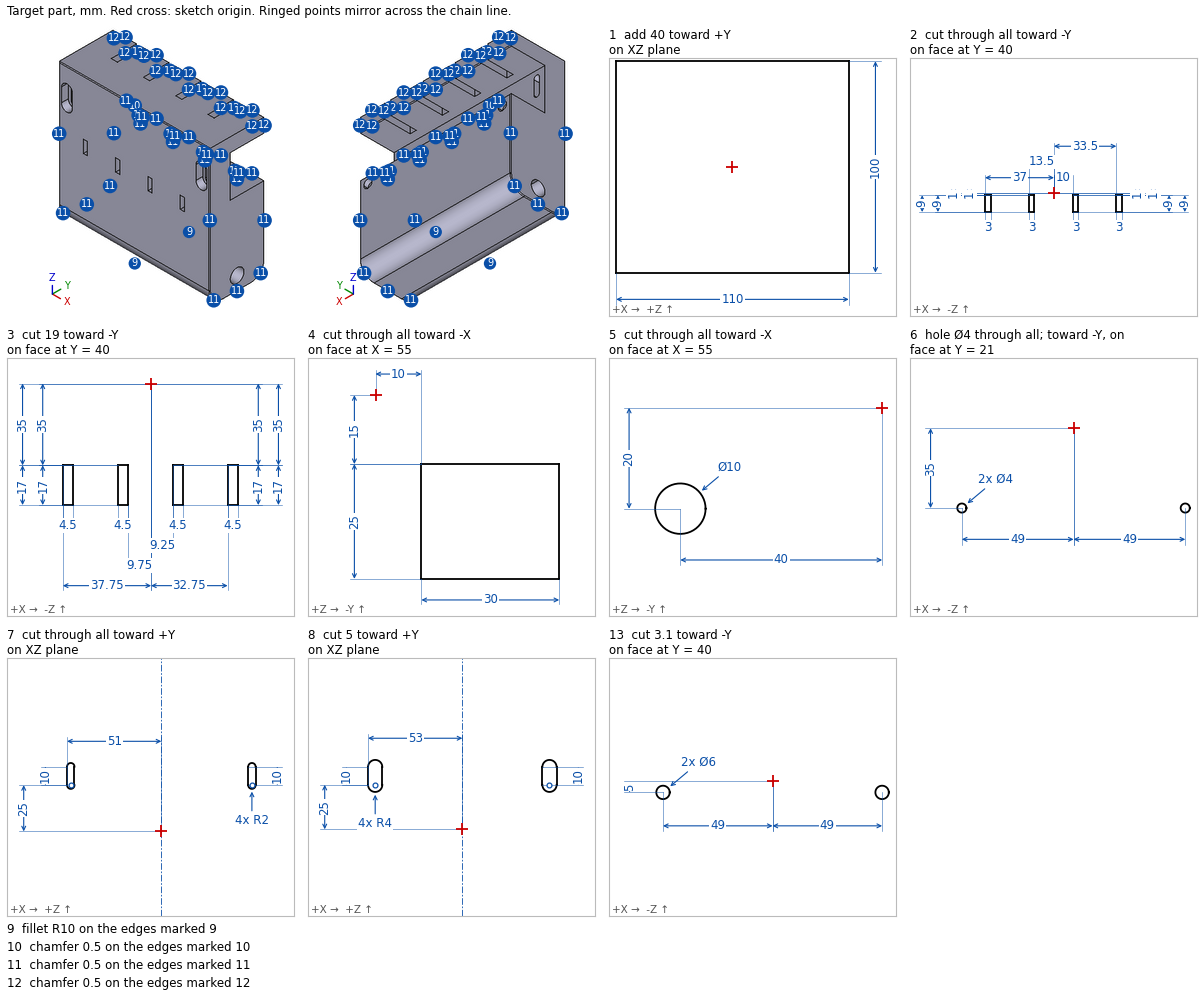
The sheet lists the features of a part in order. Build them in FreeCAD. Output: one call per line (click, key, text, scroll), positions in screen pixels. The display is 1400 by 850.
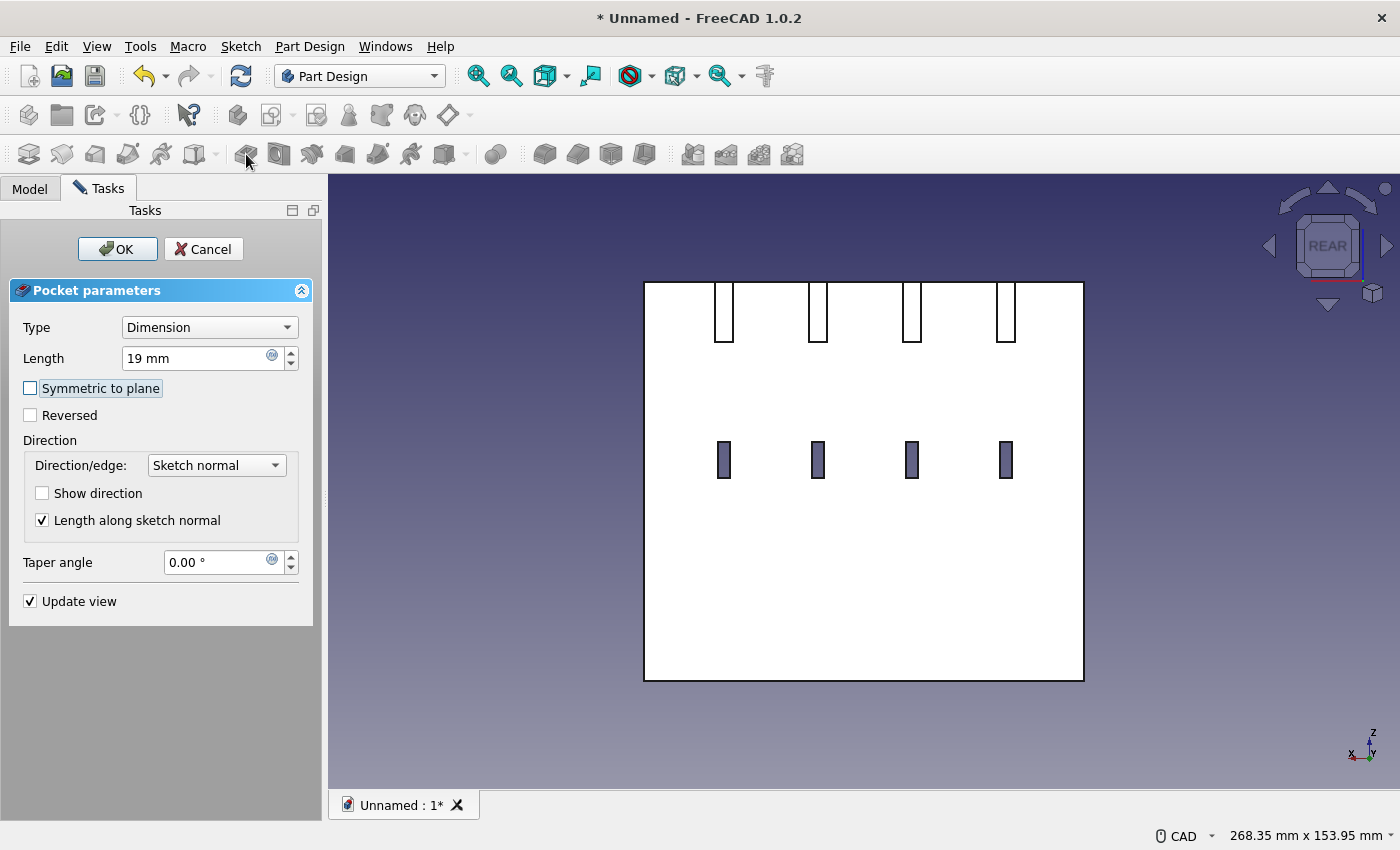
click(118, 249)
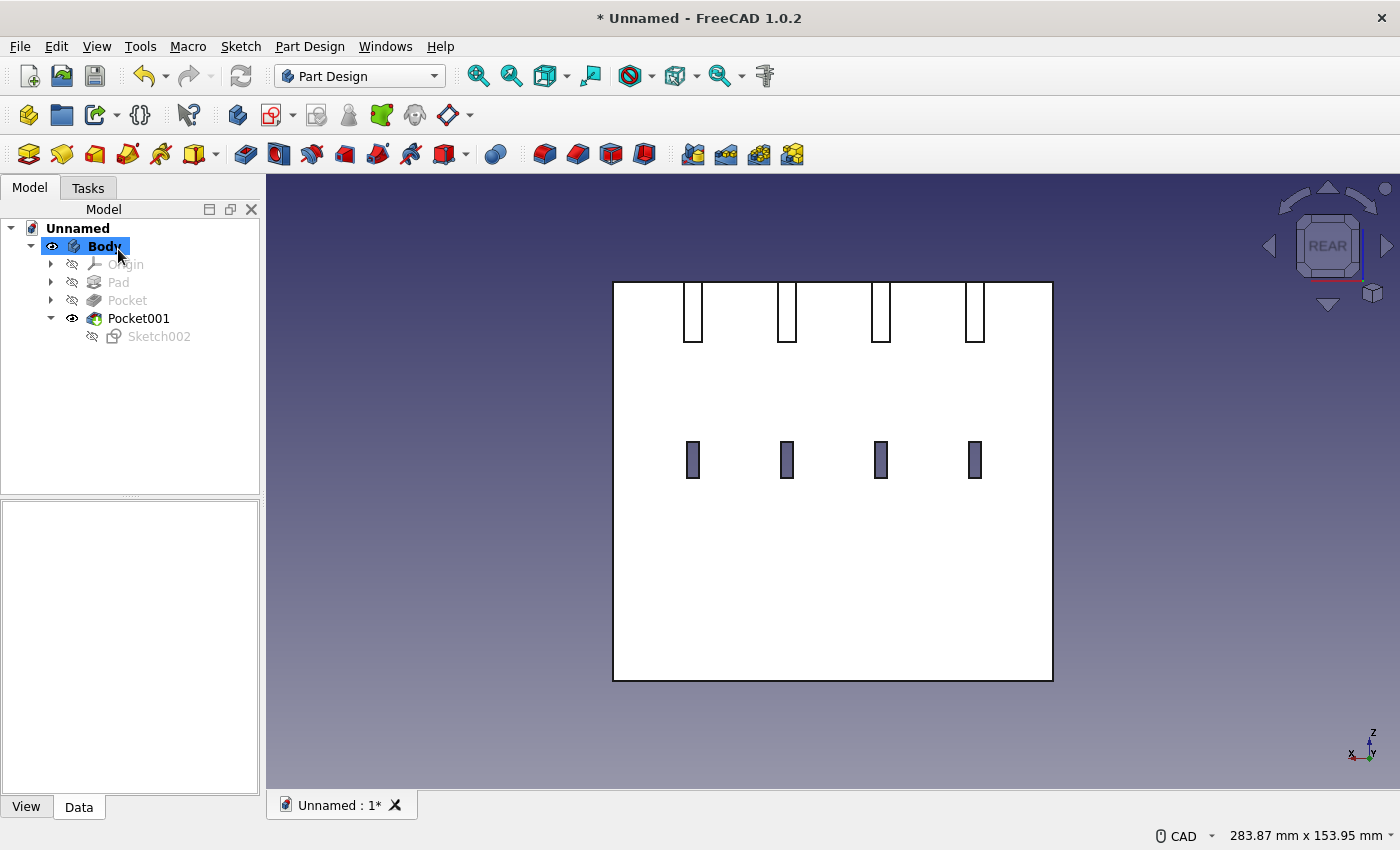
key(0)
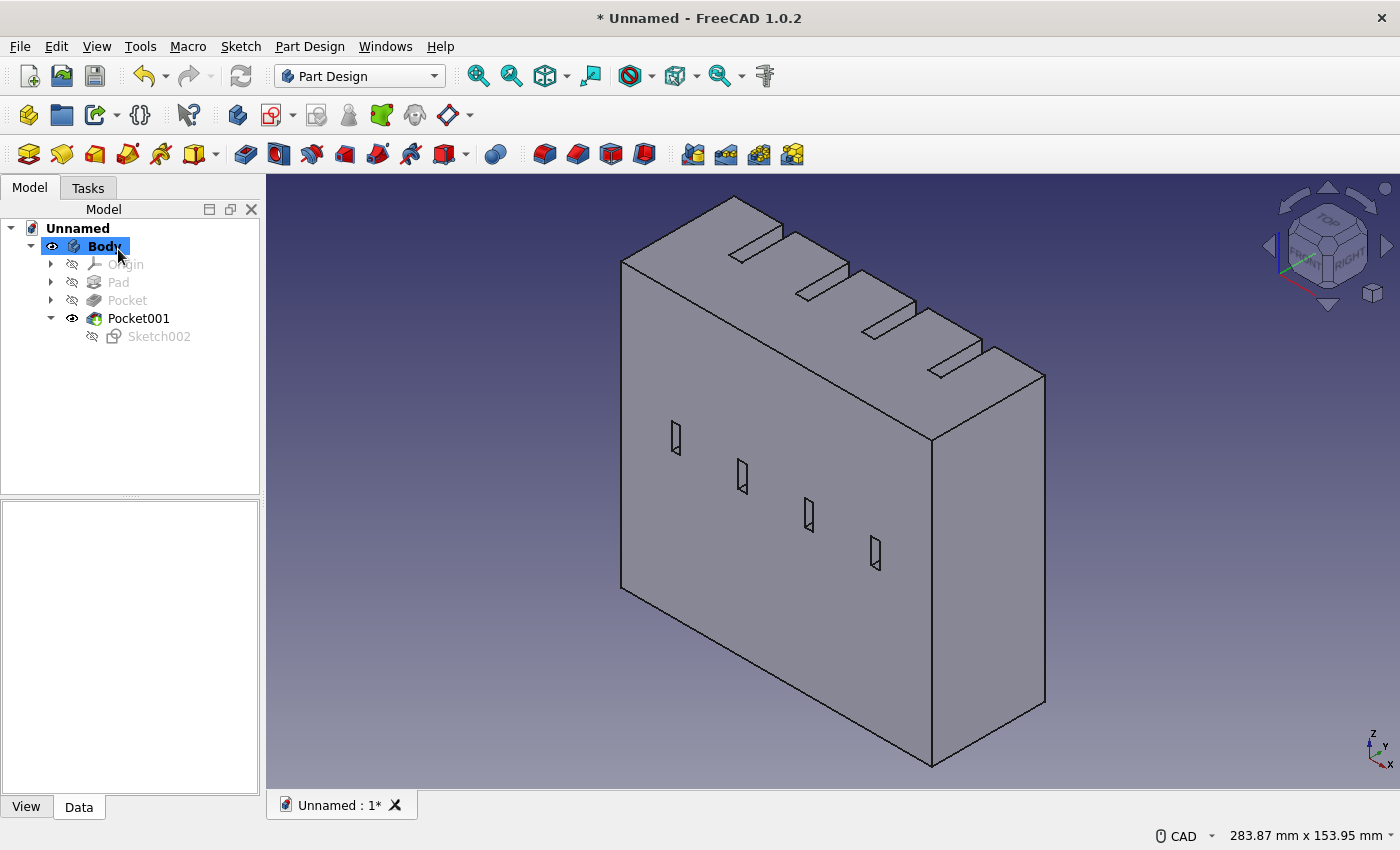
click(988, 570)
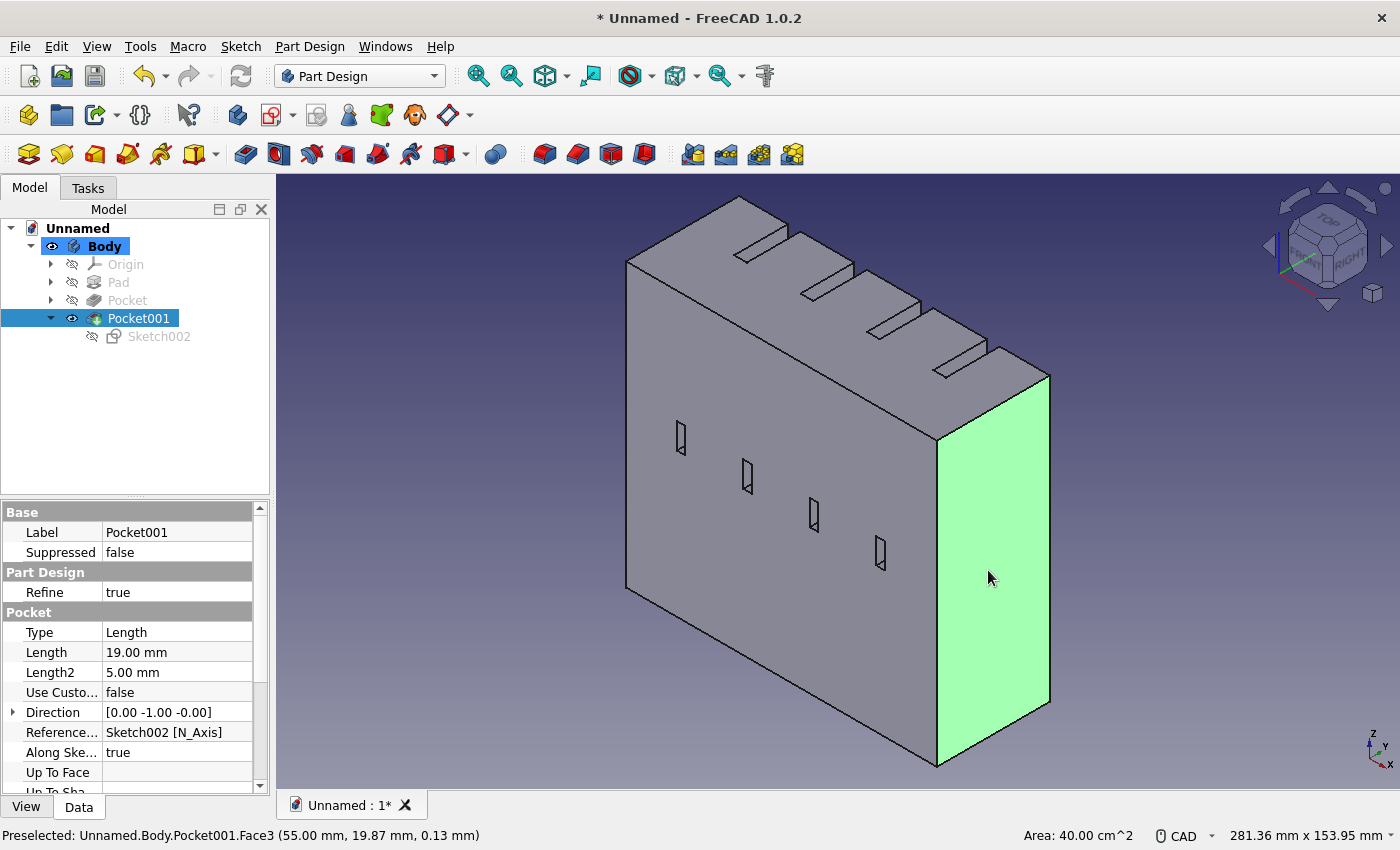
click(270, 116)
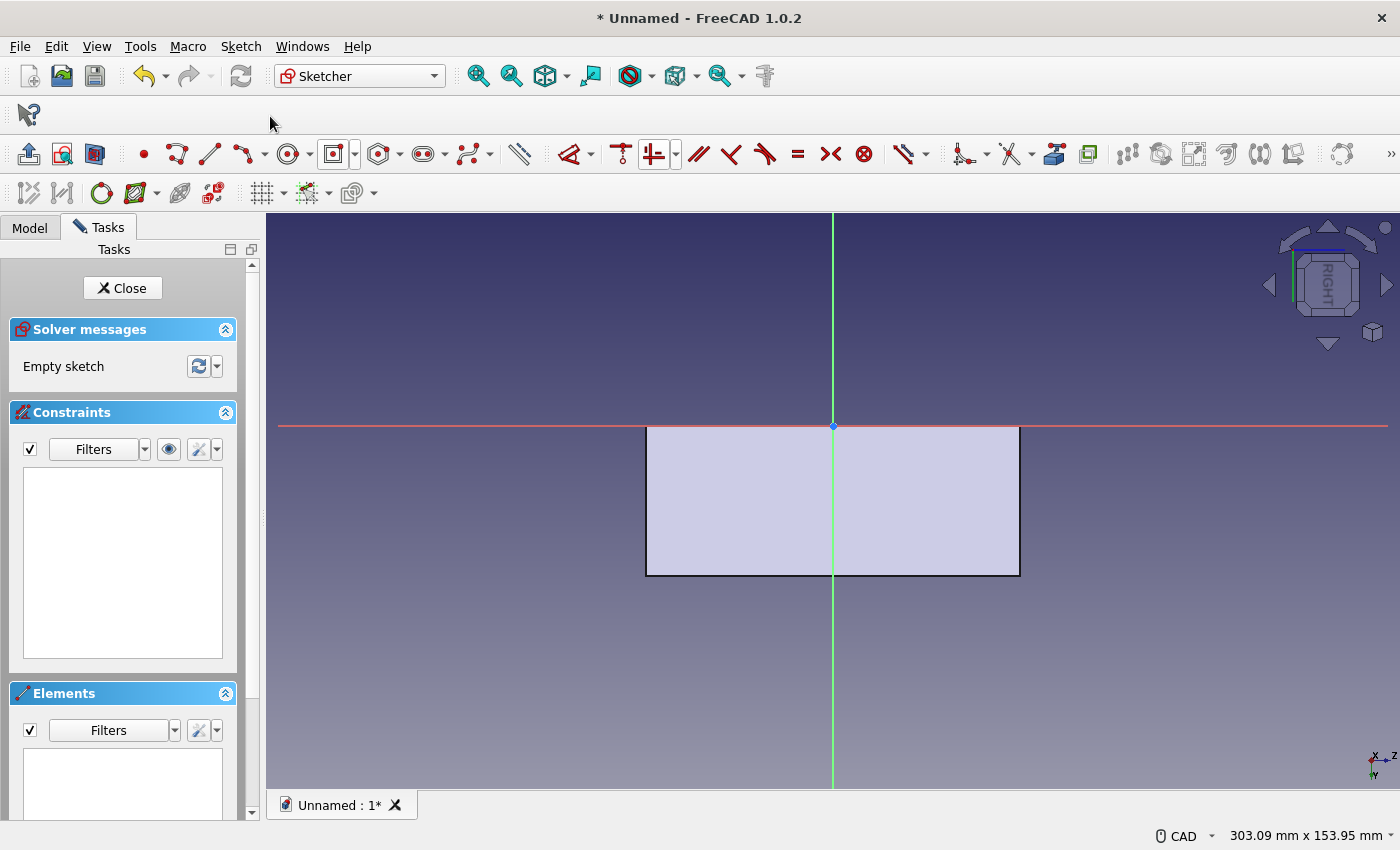
scroll(1025, 501, up, 4)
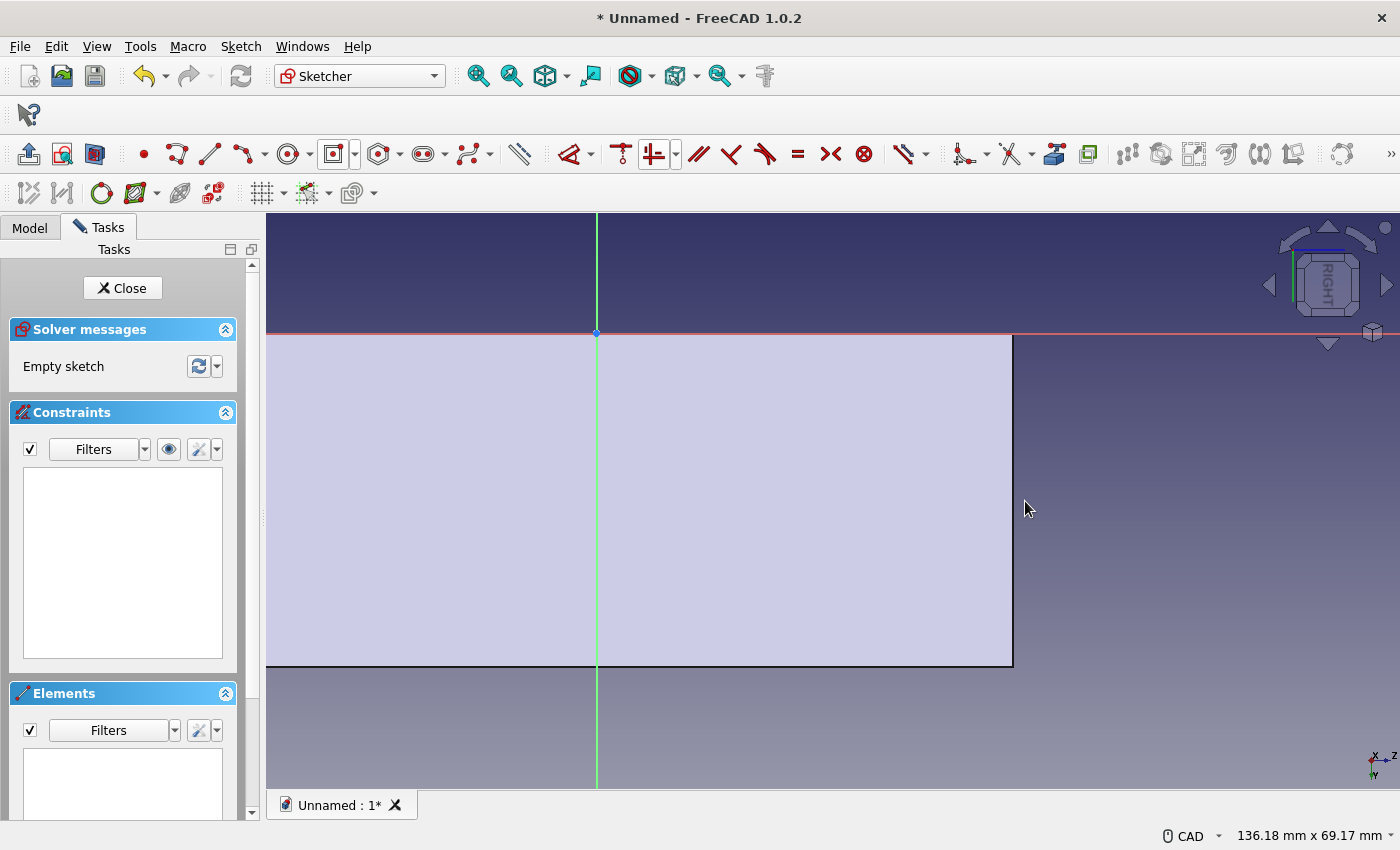
key(g)
key(r)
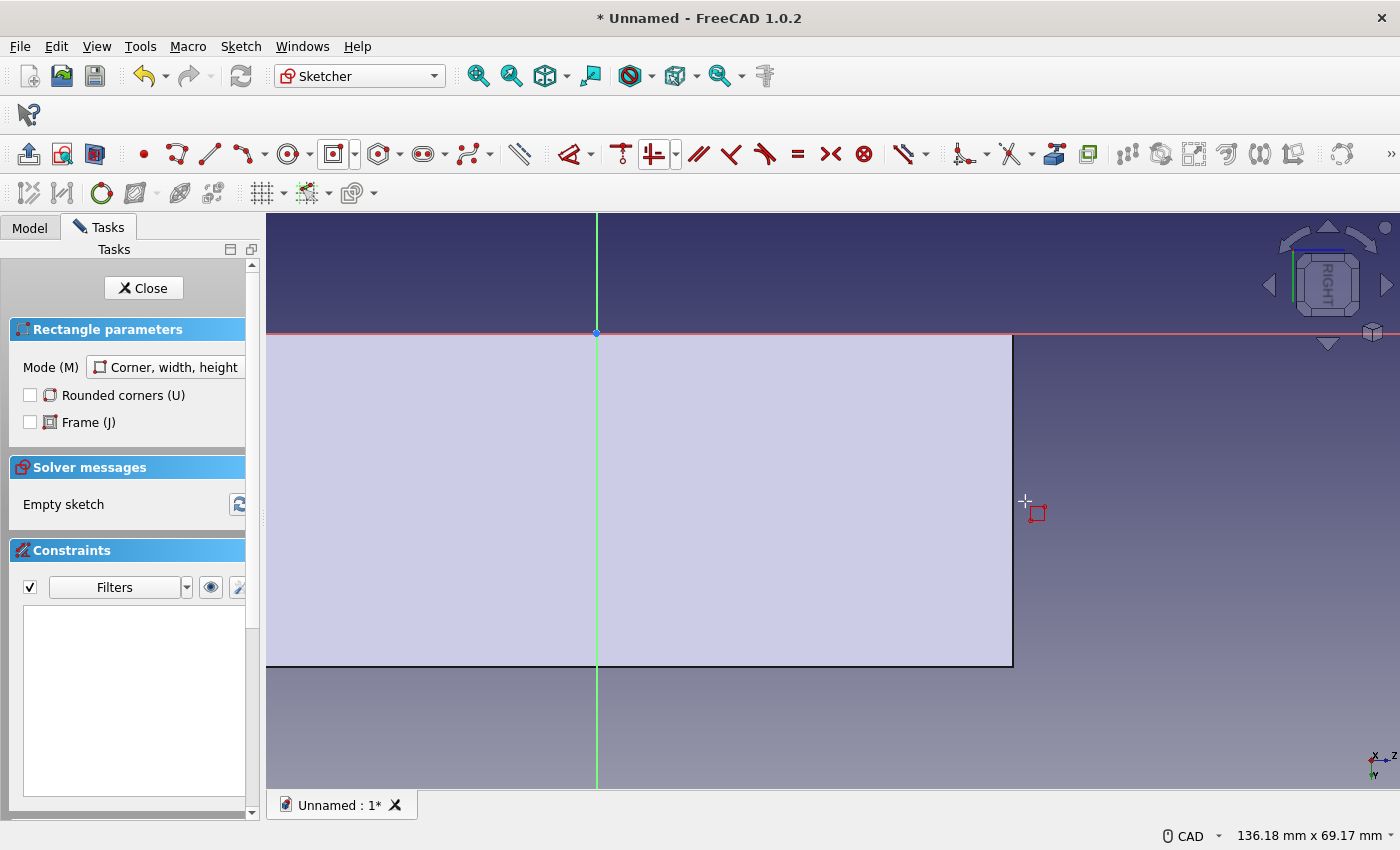
click(680, 459)
click(930, 667)
key(Escape)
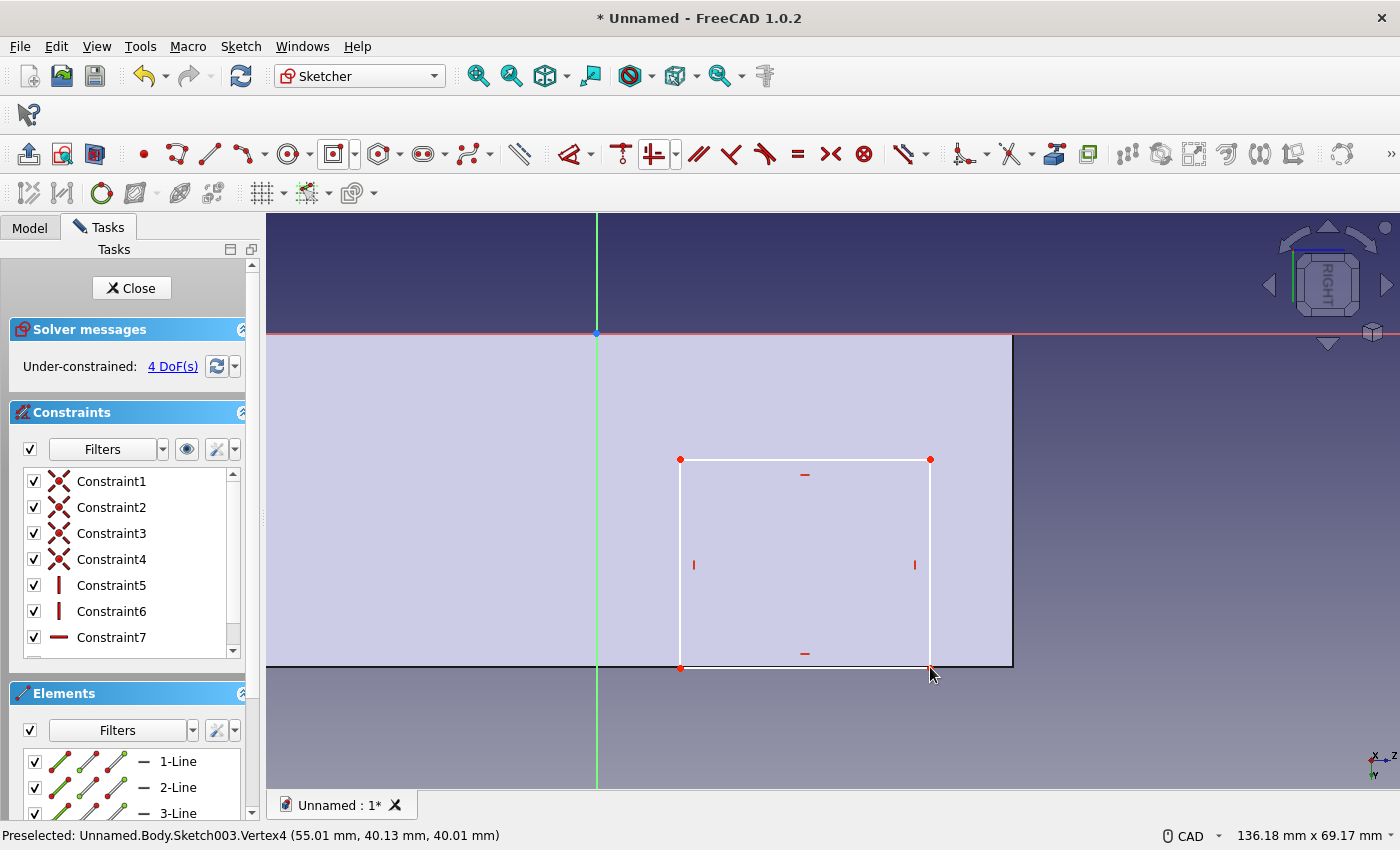
click(568, 154)